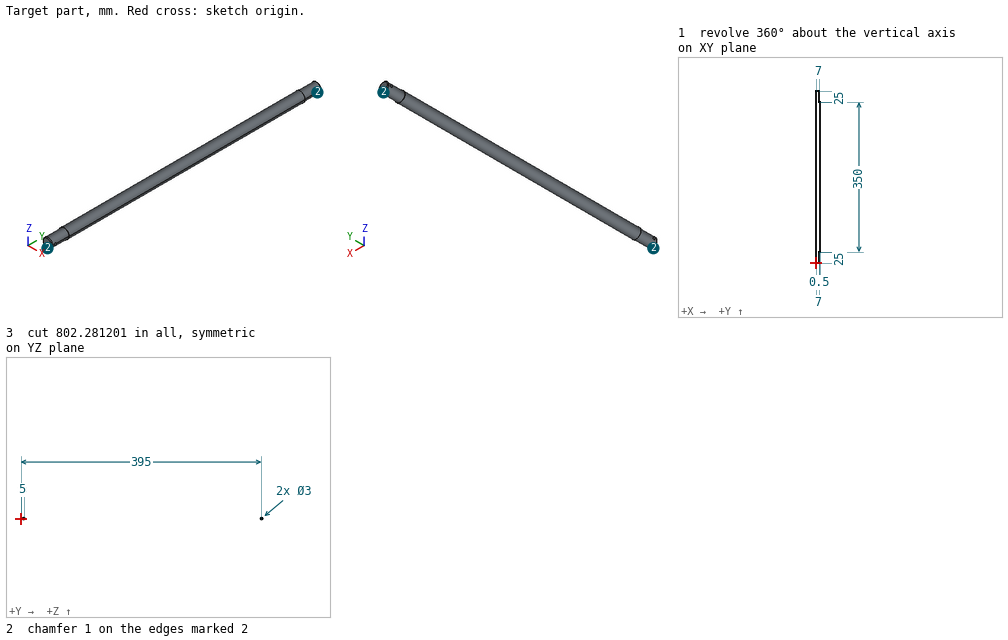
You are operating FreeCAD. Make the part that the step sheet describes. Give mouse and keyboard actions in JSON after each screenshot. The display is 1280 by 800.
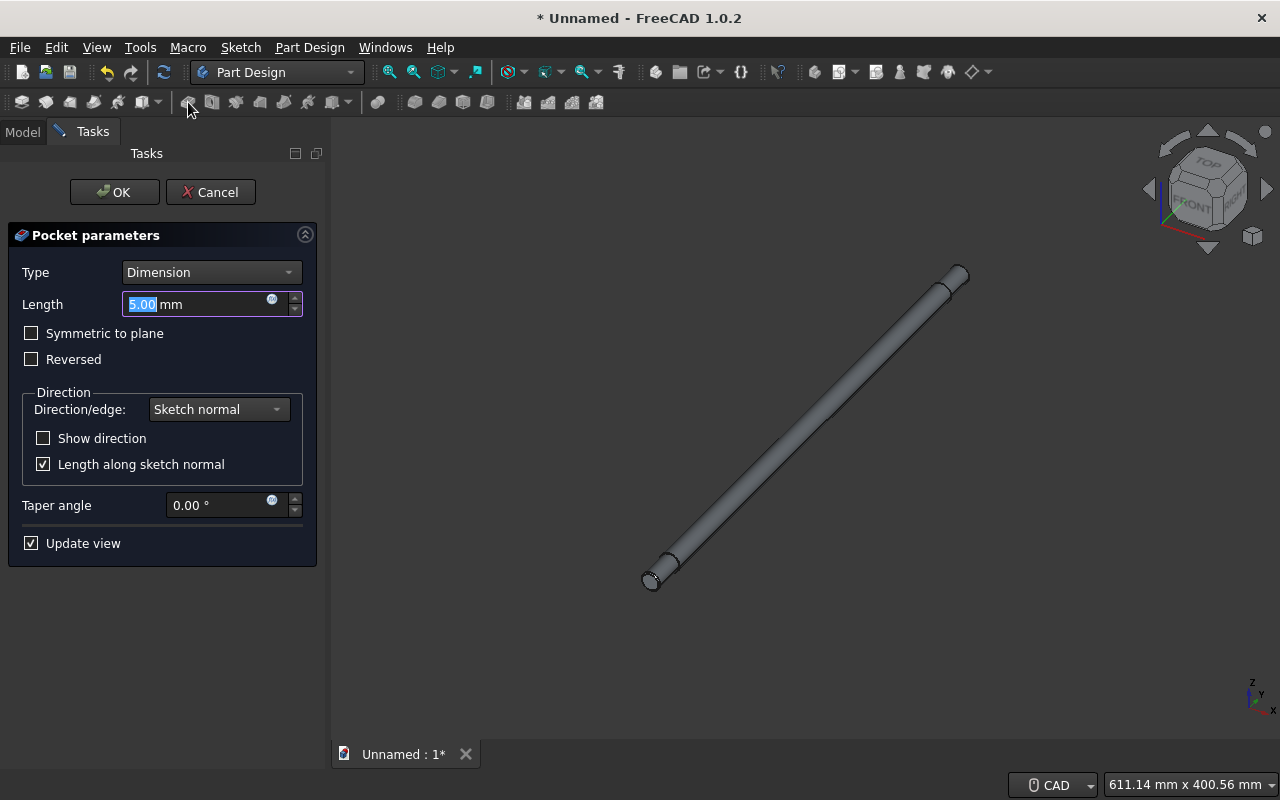
{"action": "type", "text": "802.281201"}
{"action": "key", "text": "Tab"}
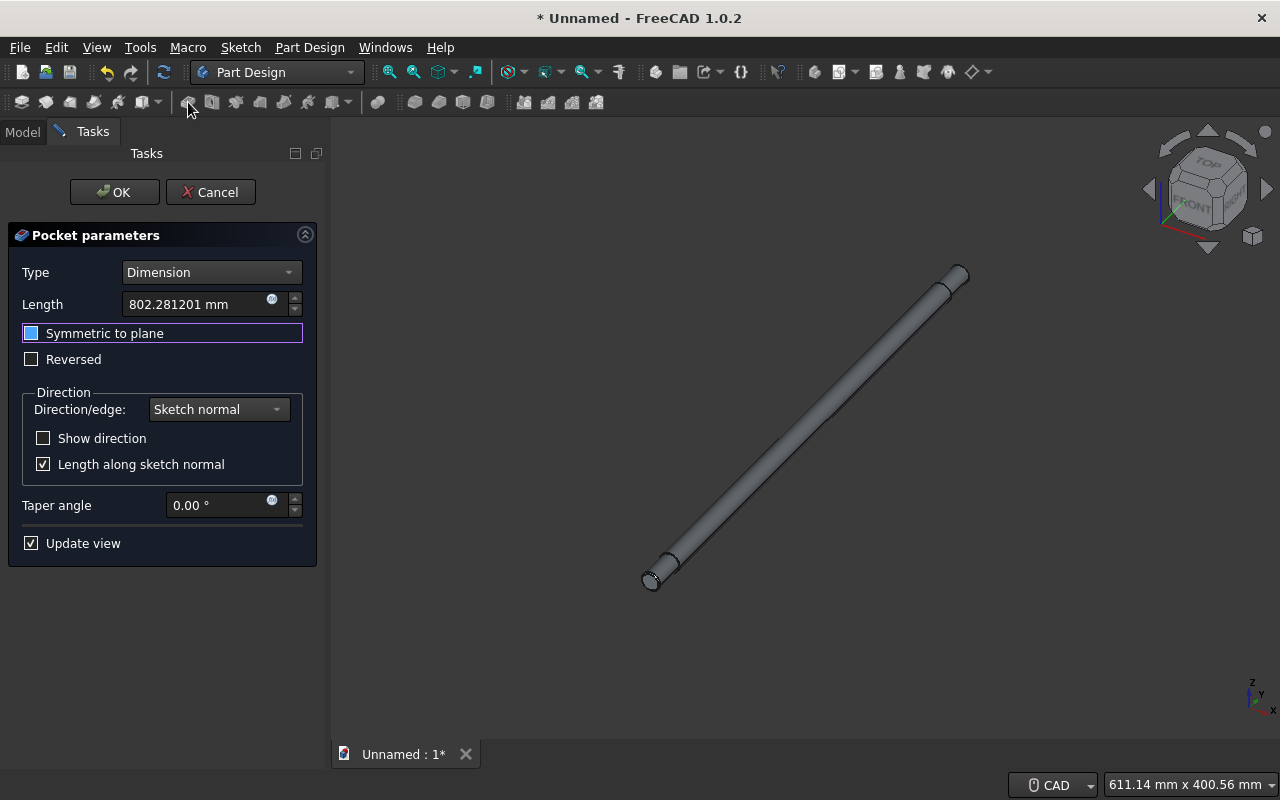
{"action": "left_click", "coordinate": [30, 333]}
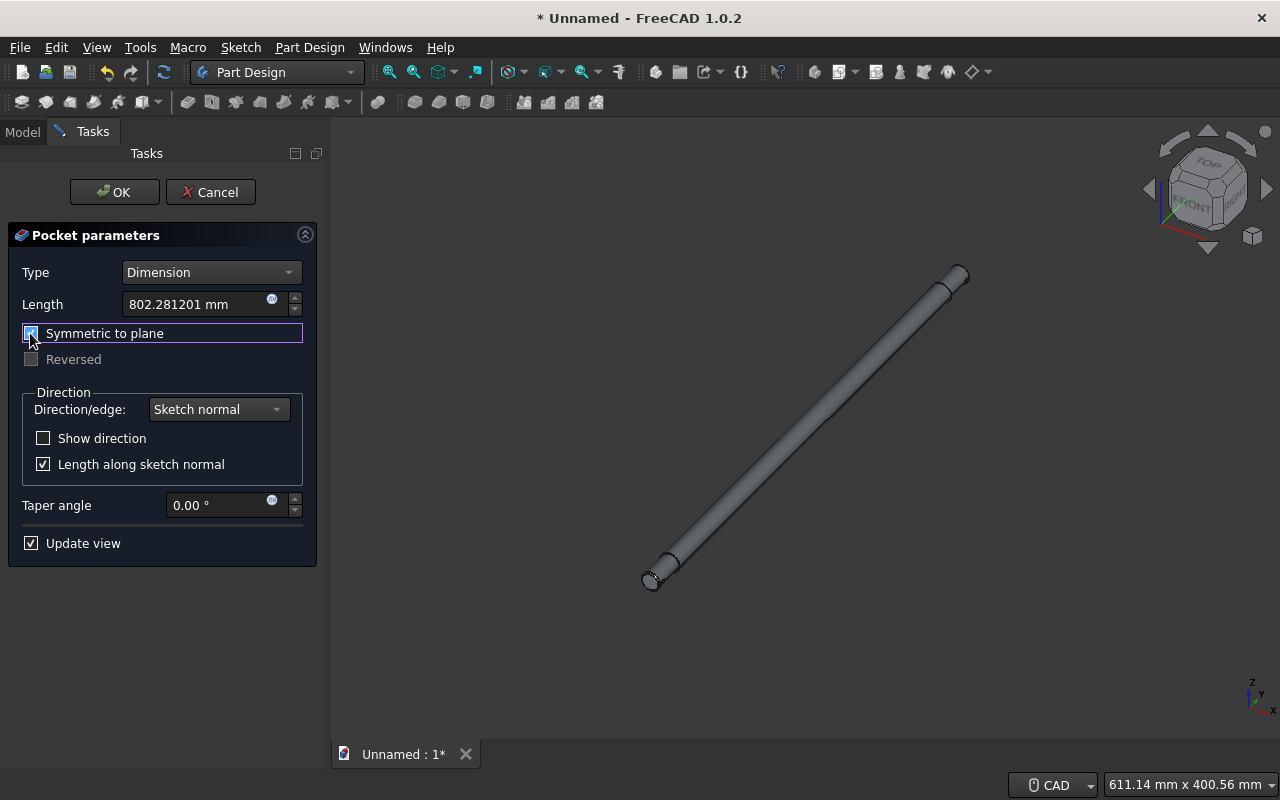
{"action": "left_click", "coordinate": [115, 192]}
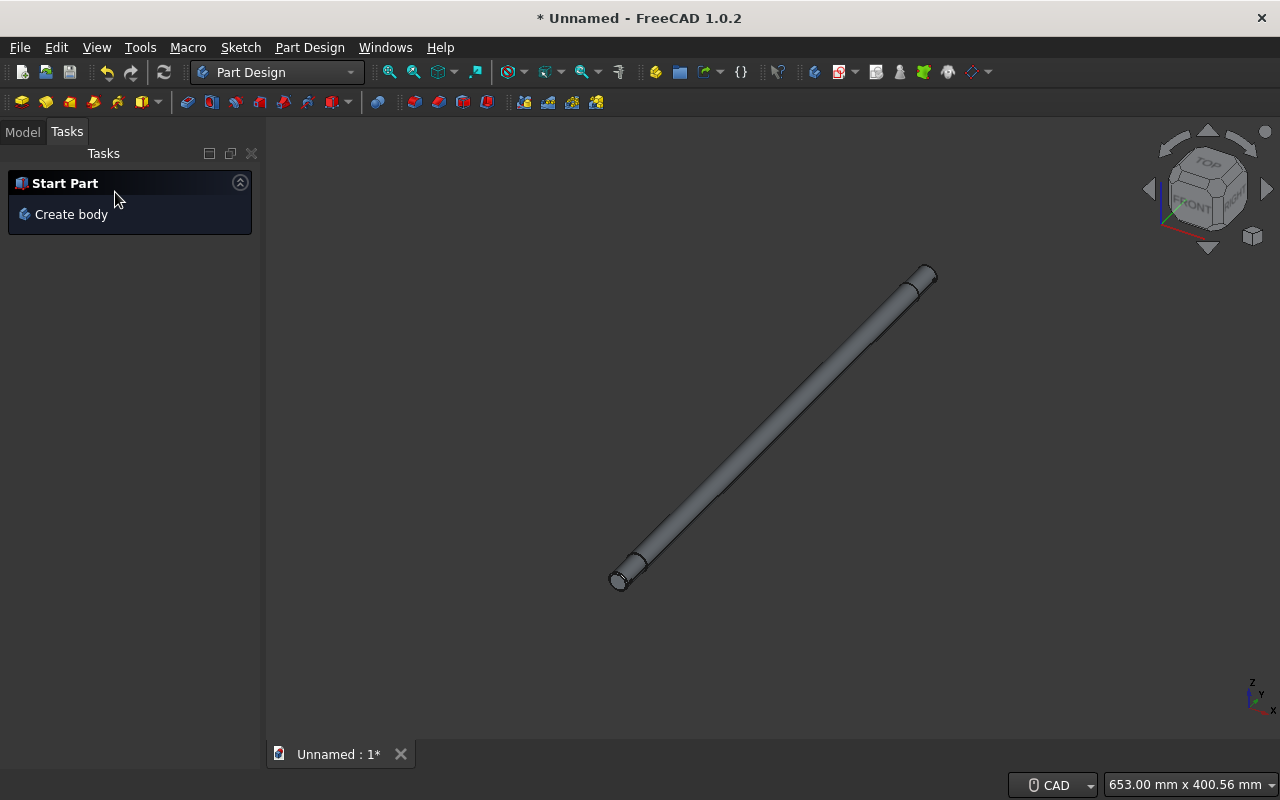
{"action": "key", "text": "0"}